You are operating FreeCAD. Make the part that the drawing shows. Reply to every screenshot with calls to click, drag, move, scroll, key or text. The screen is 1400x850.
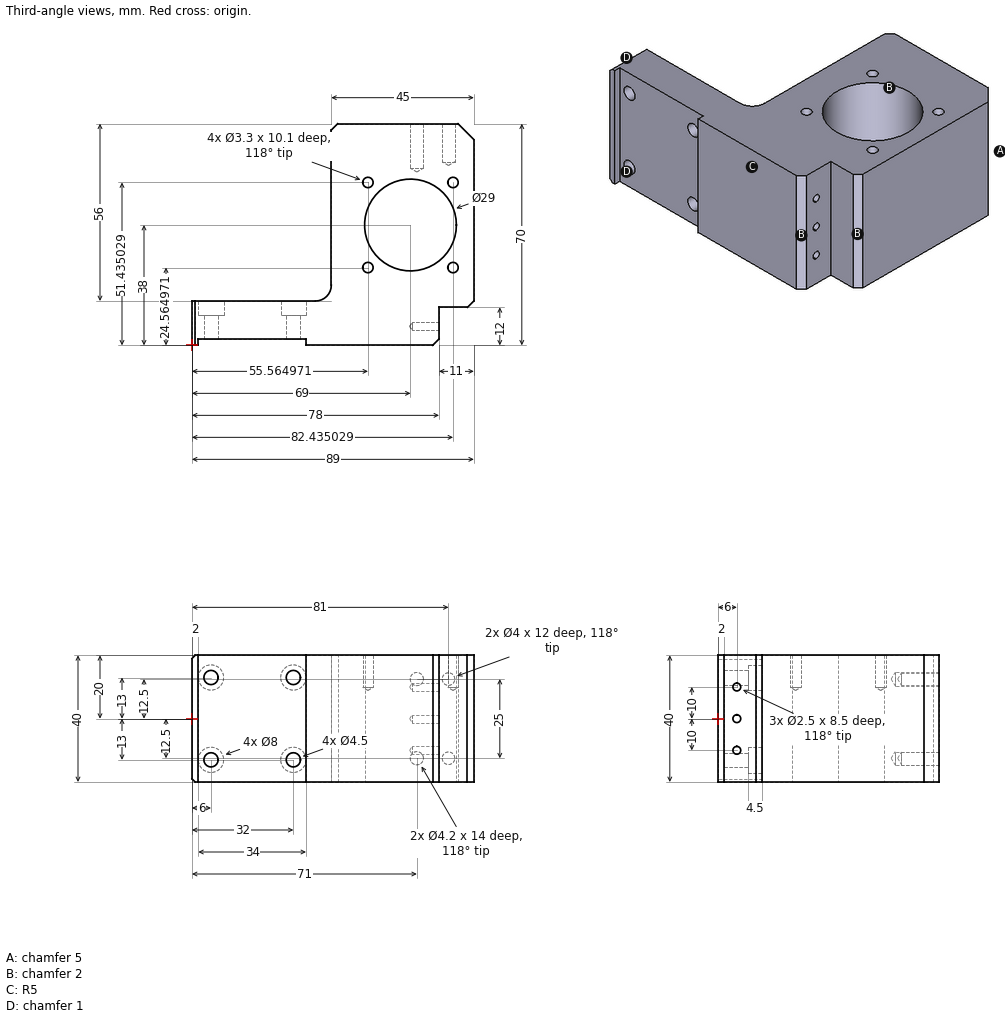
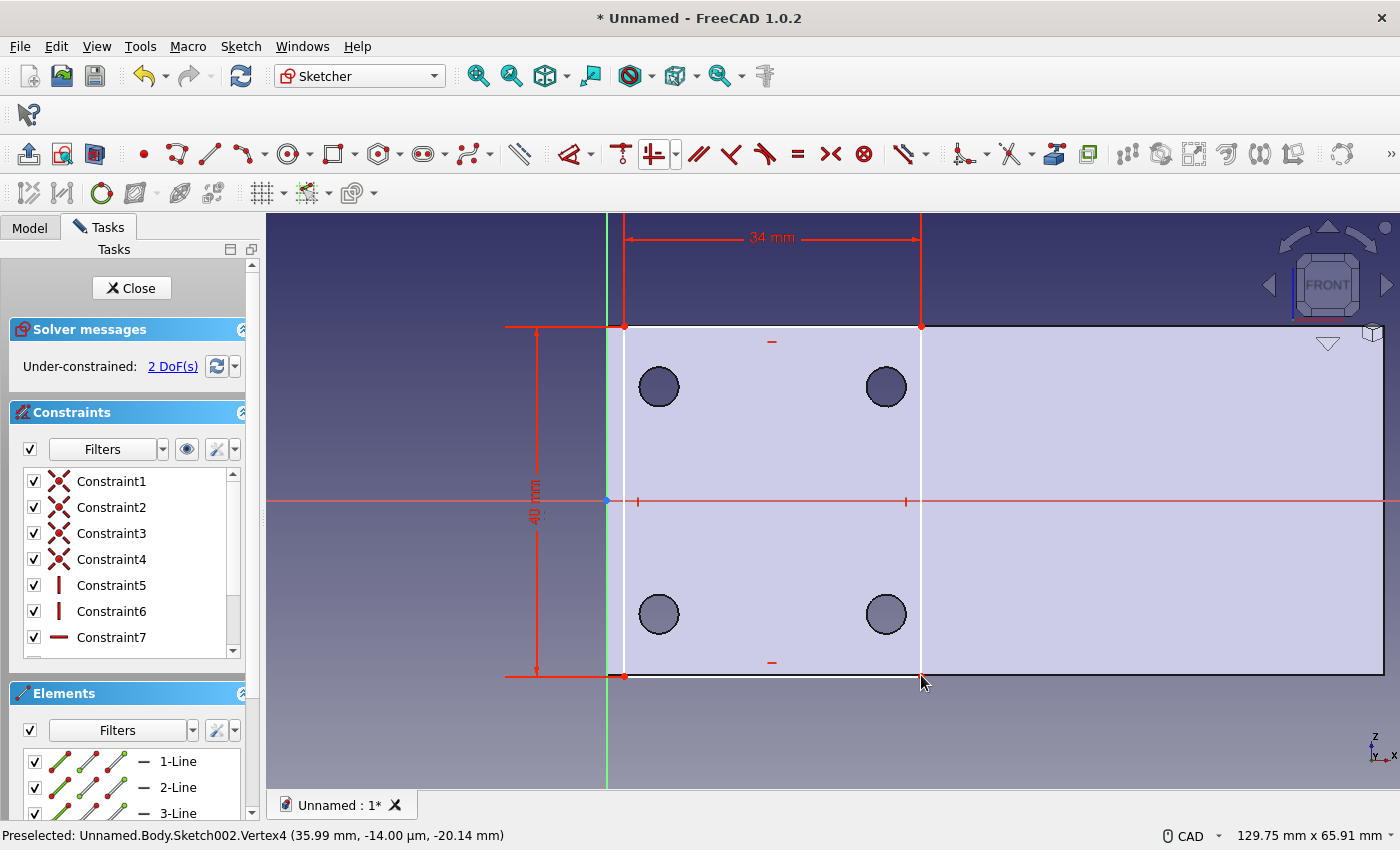
click(568, 154)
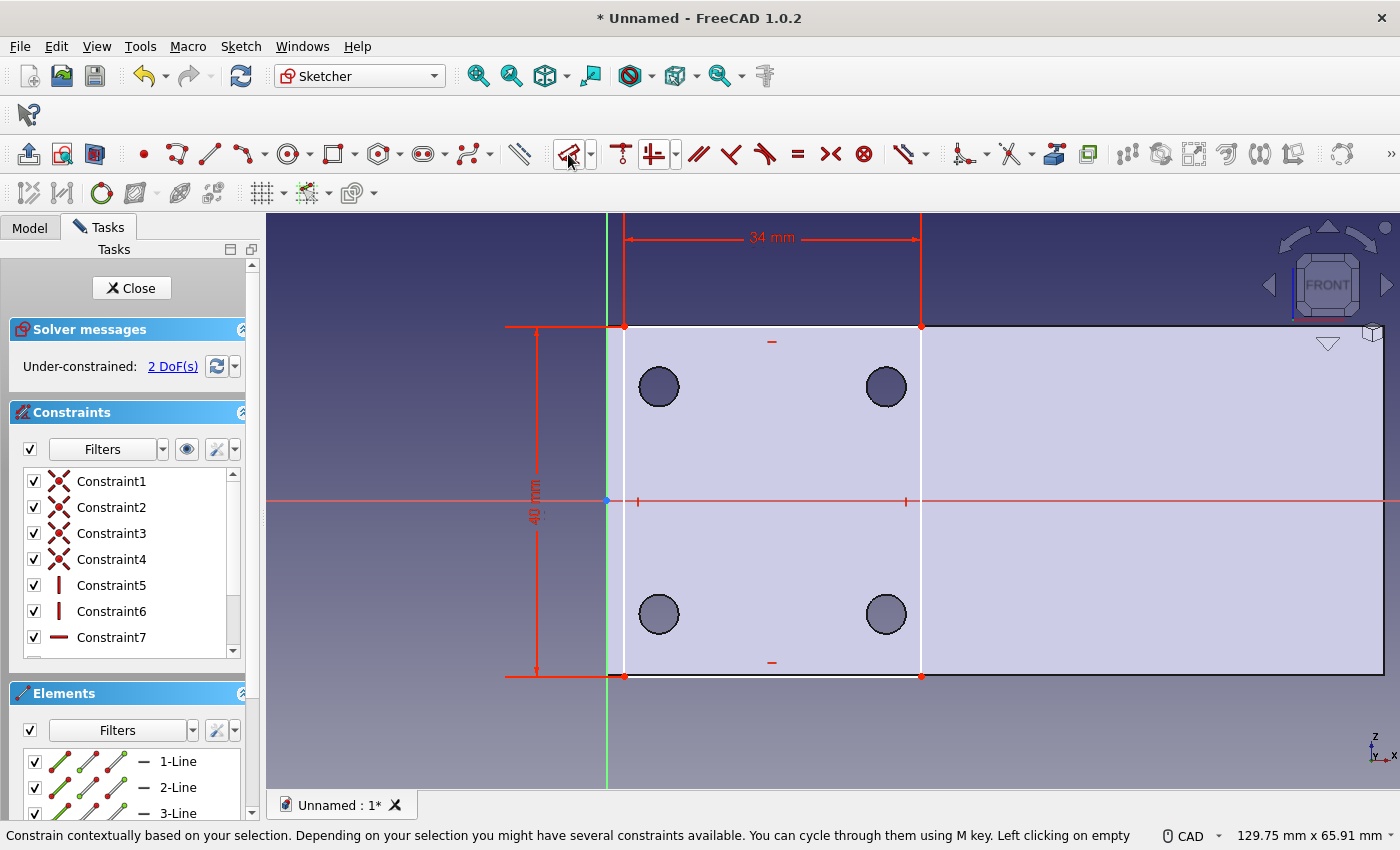
scroll(624, 327, up, 5)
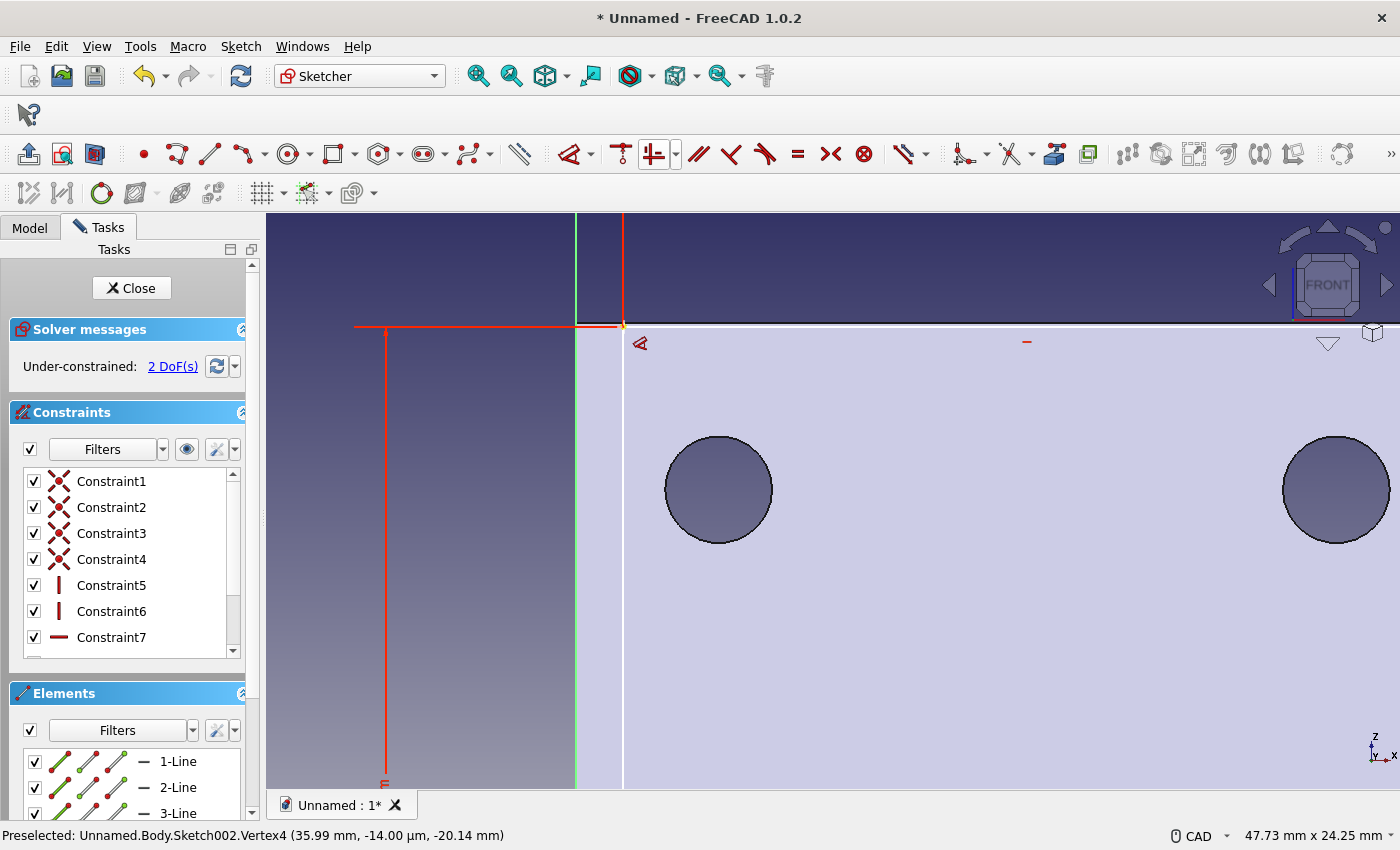
click(623, 327)
click(600, 293)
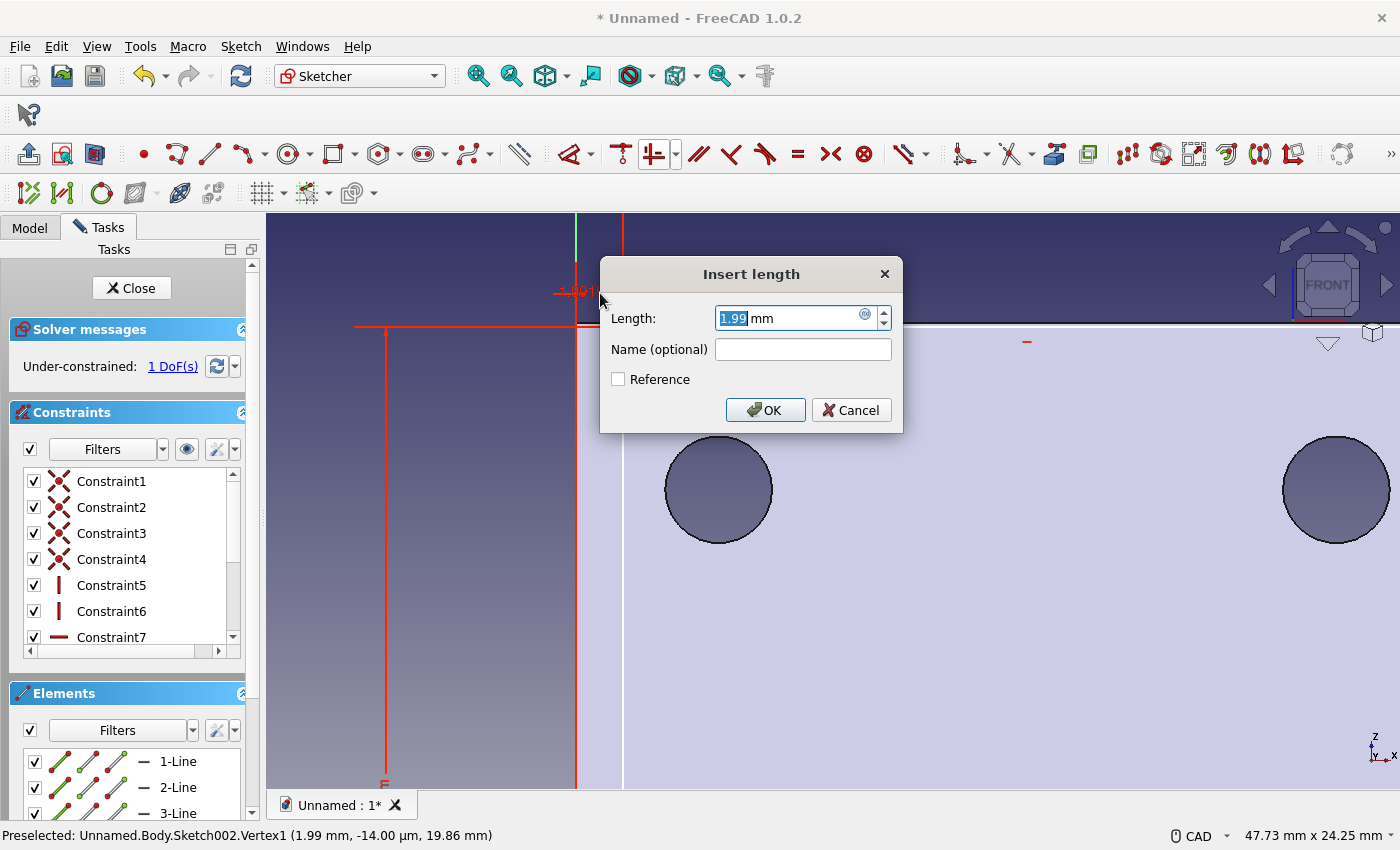
text(2)
key(Return)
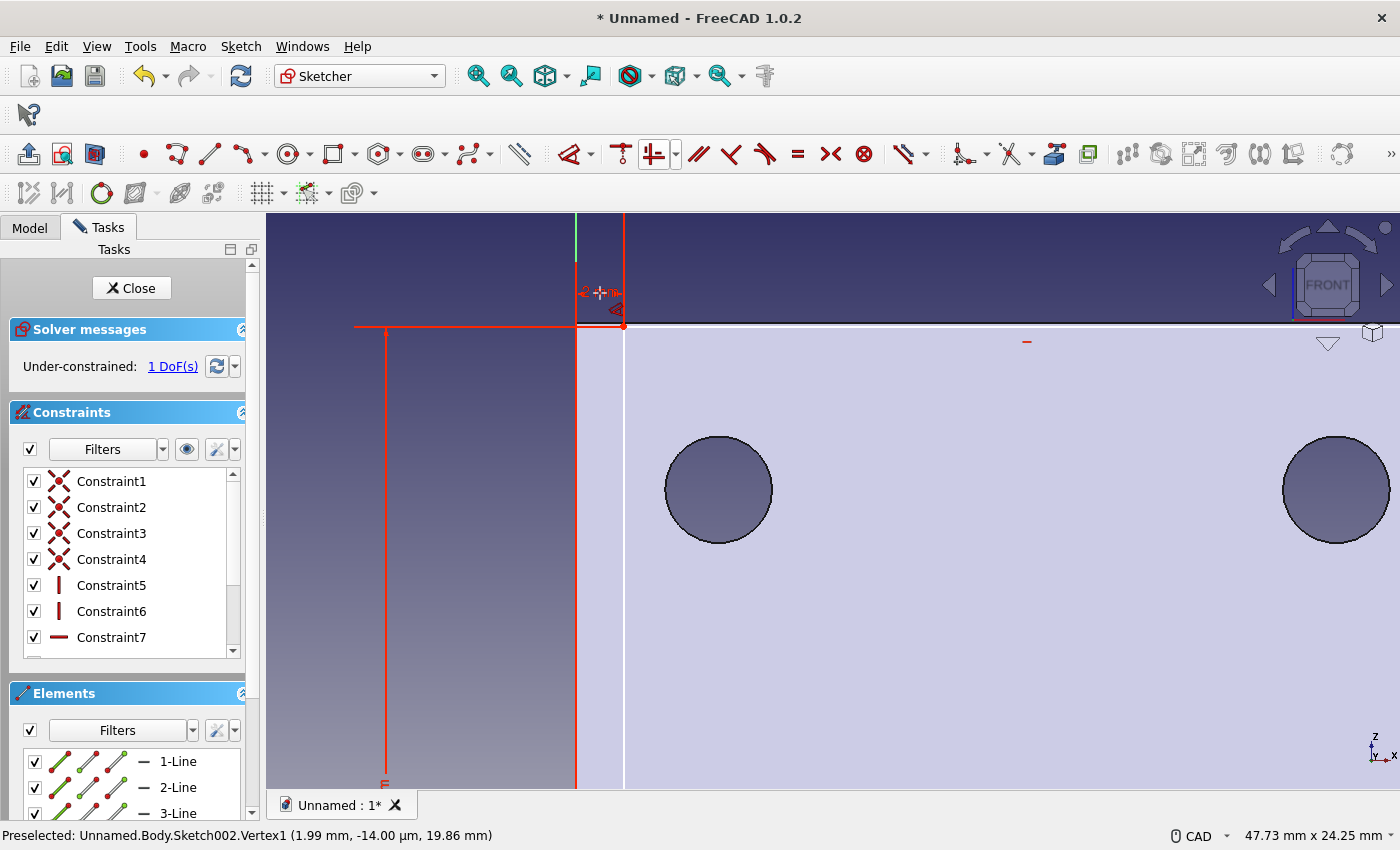
click(624, 327)
click(542, 544)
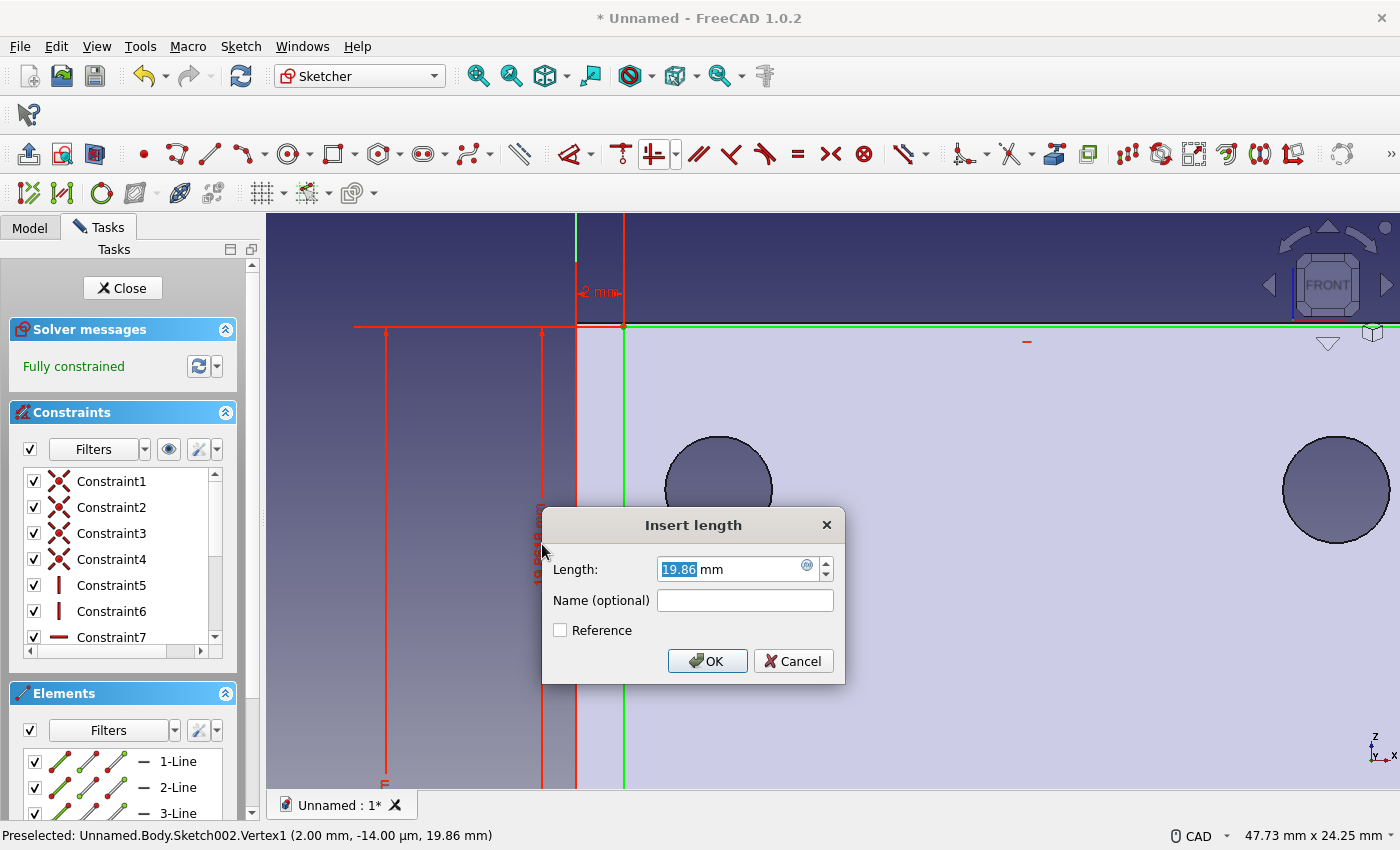
text(20)
key(Return)
key(Escape)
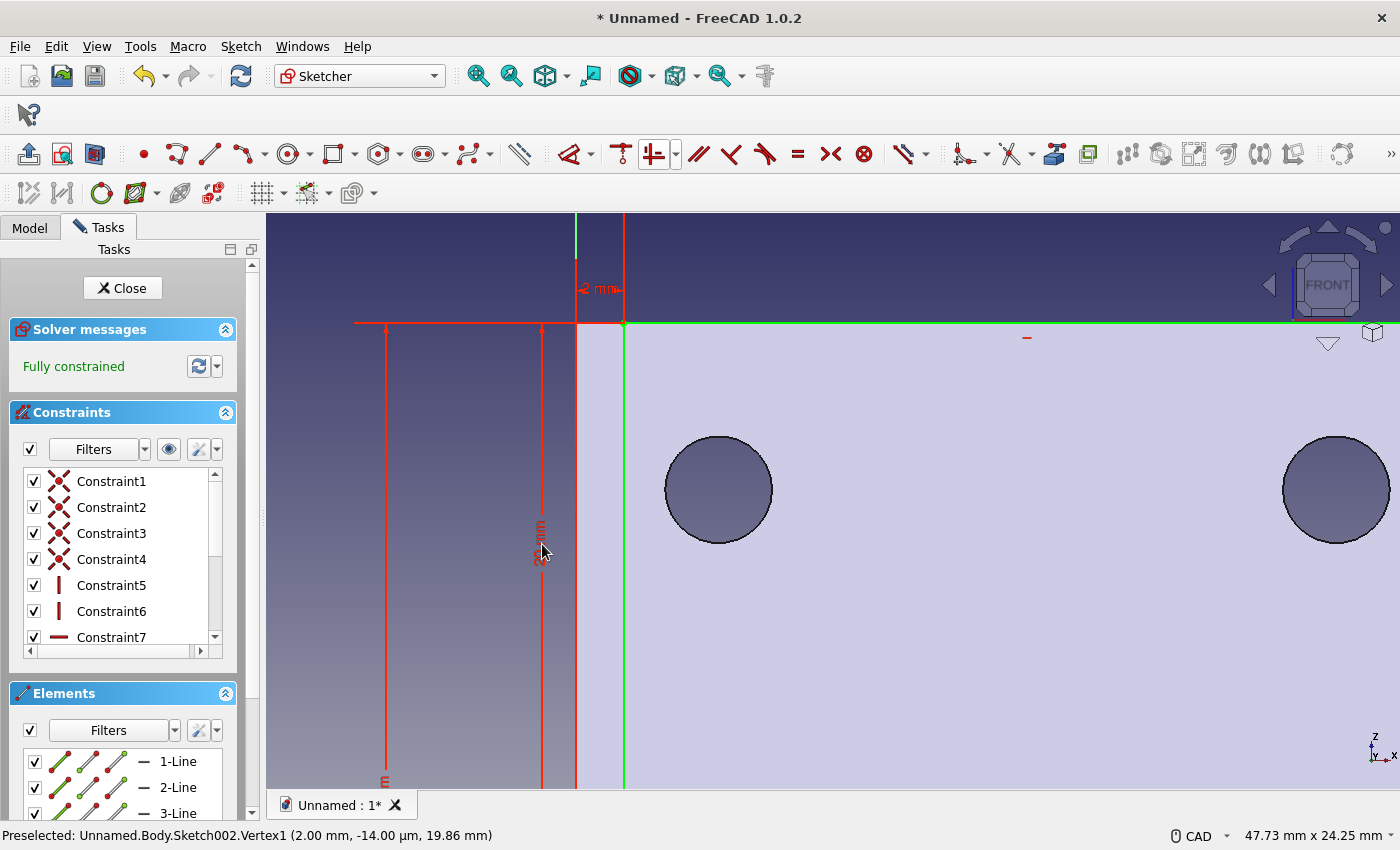
click(123, 288)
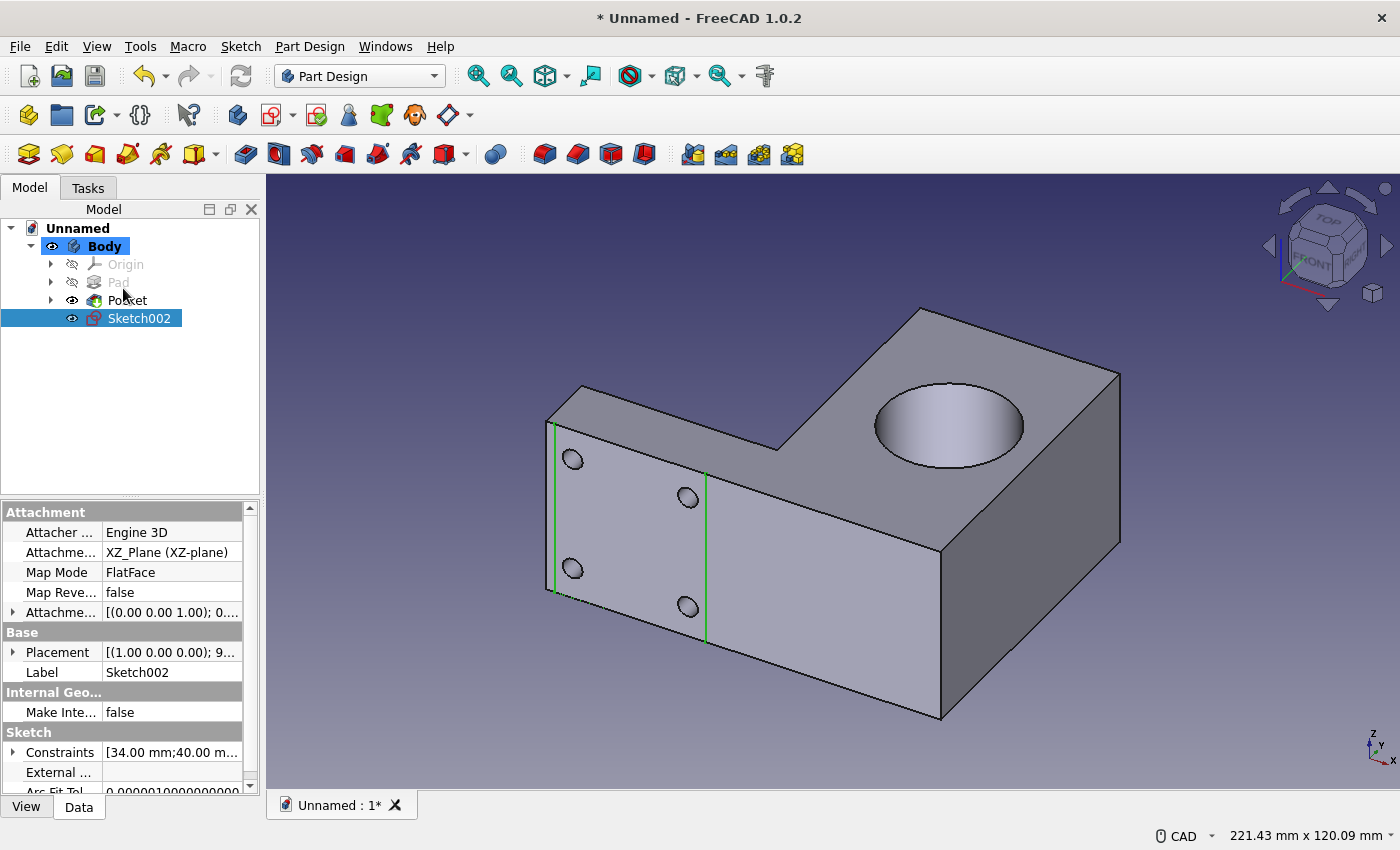
click(246, 154)